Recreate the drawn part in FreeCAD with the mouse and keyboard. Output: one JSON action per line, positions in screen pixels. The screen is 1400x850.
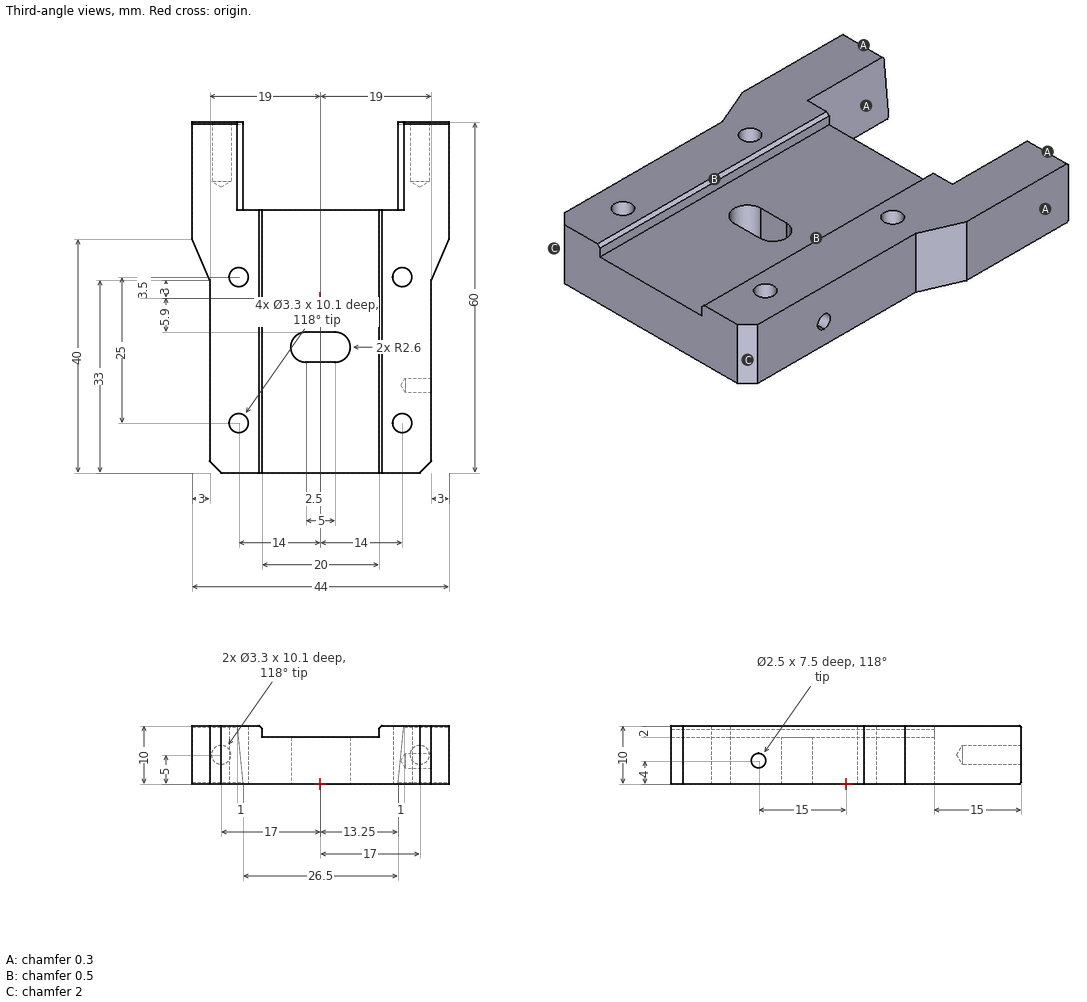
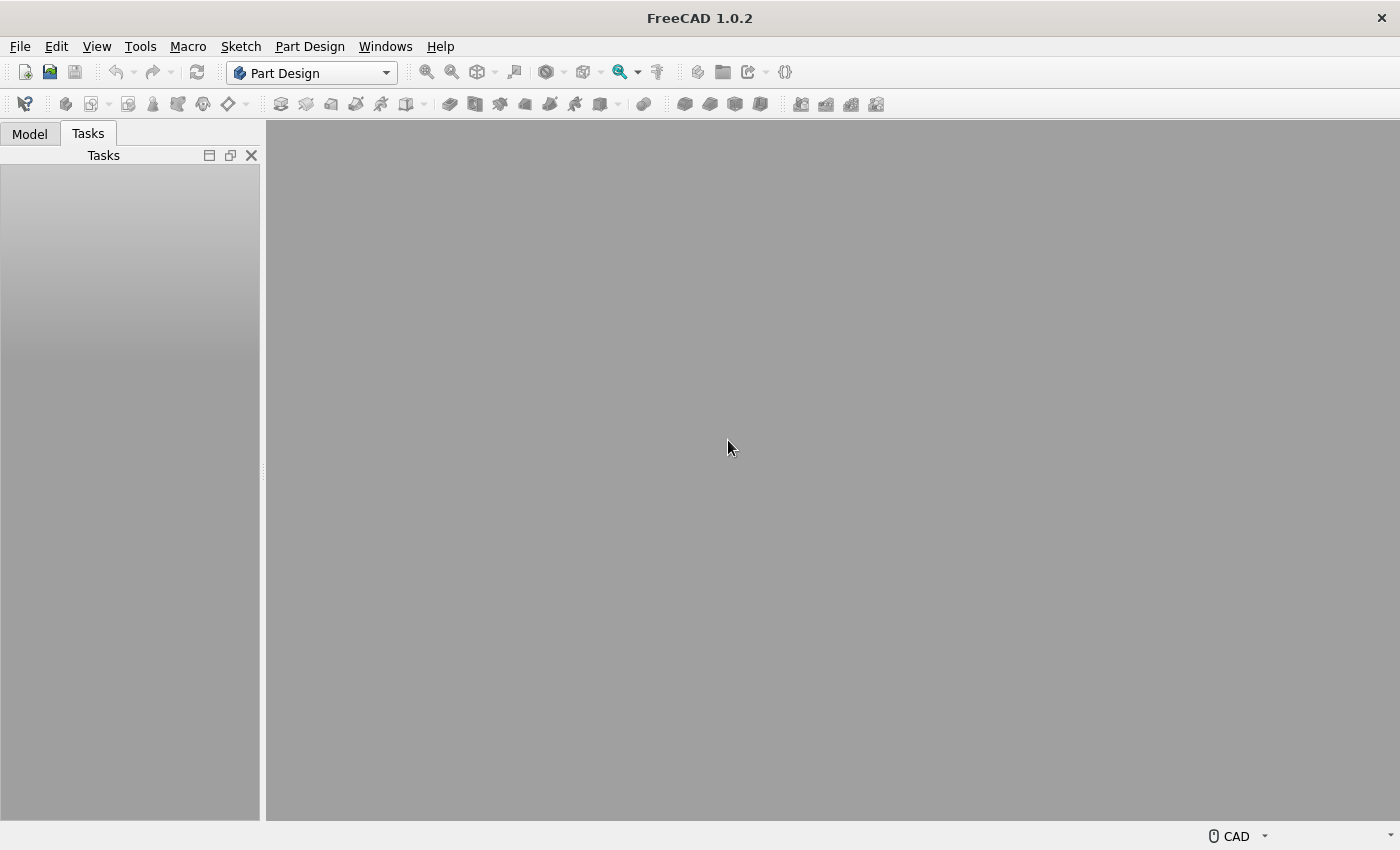
{"action": "key", "text": "ctrl+n"}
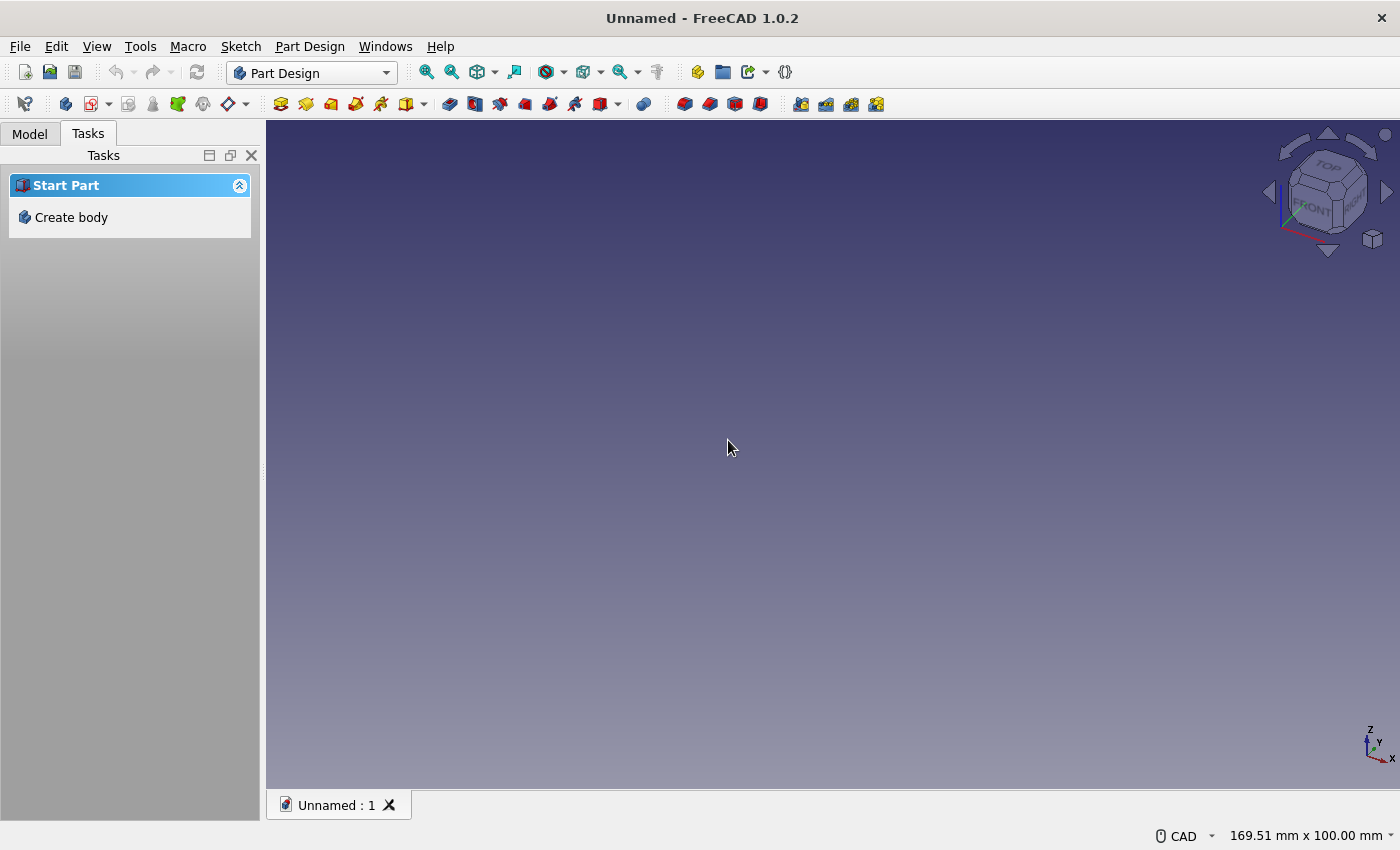
{"action": "left_click", "coordinate": [90, 104]}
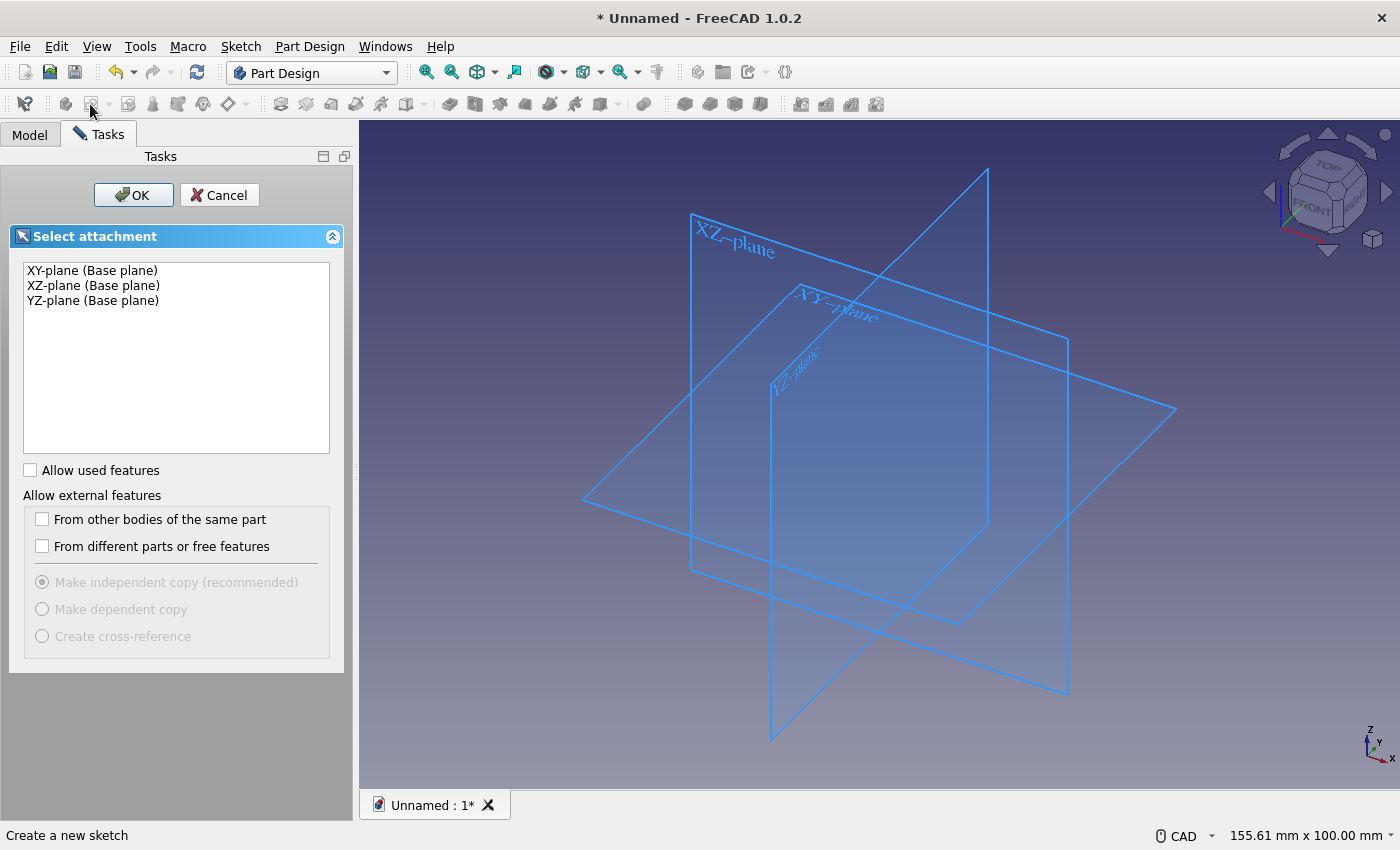
{"action": "left_click", "coordinate": [84, 270]}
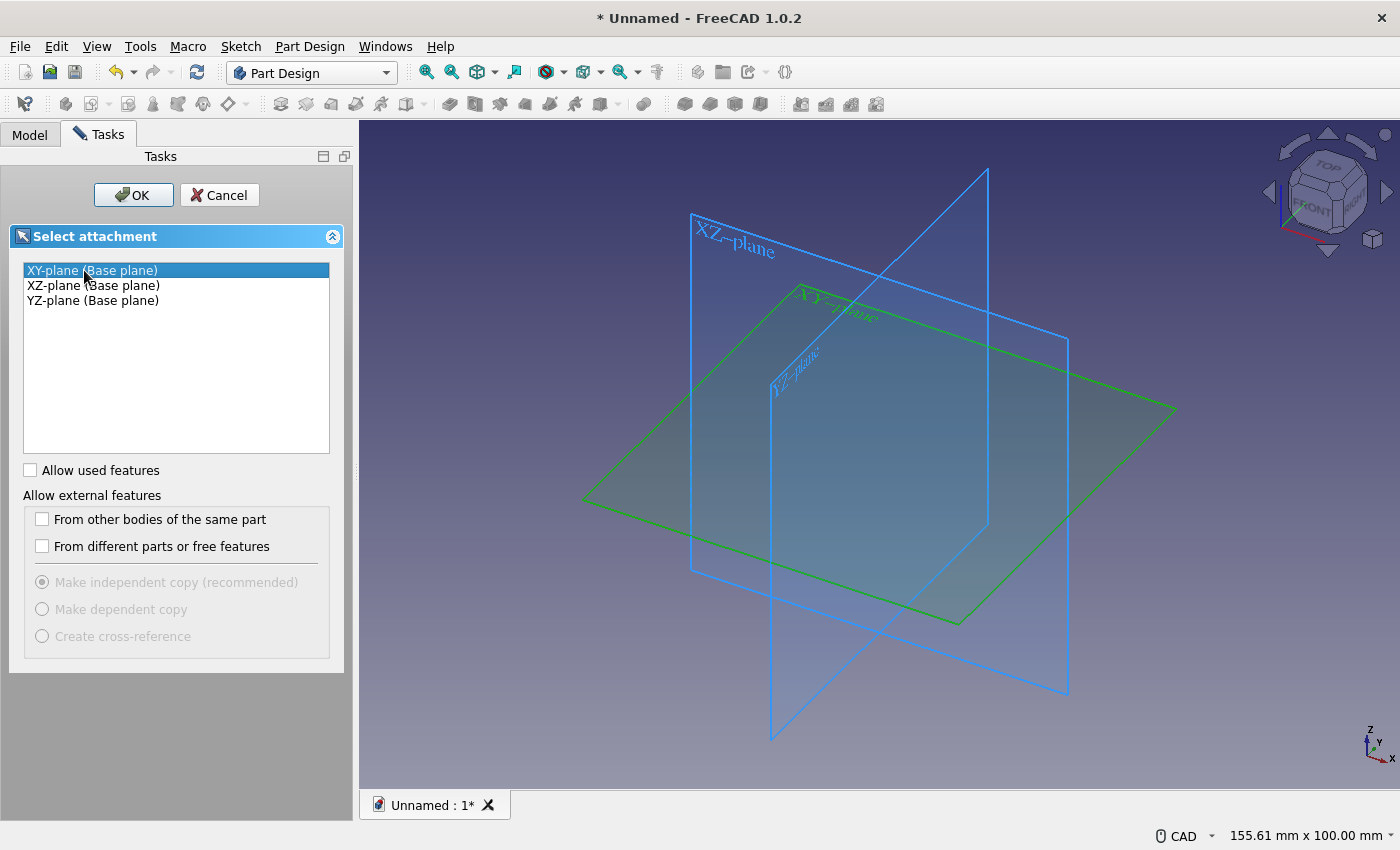
{"action": "left_click", "coordinate": [134, 195]}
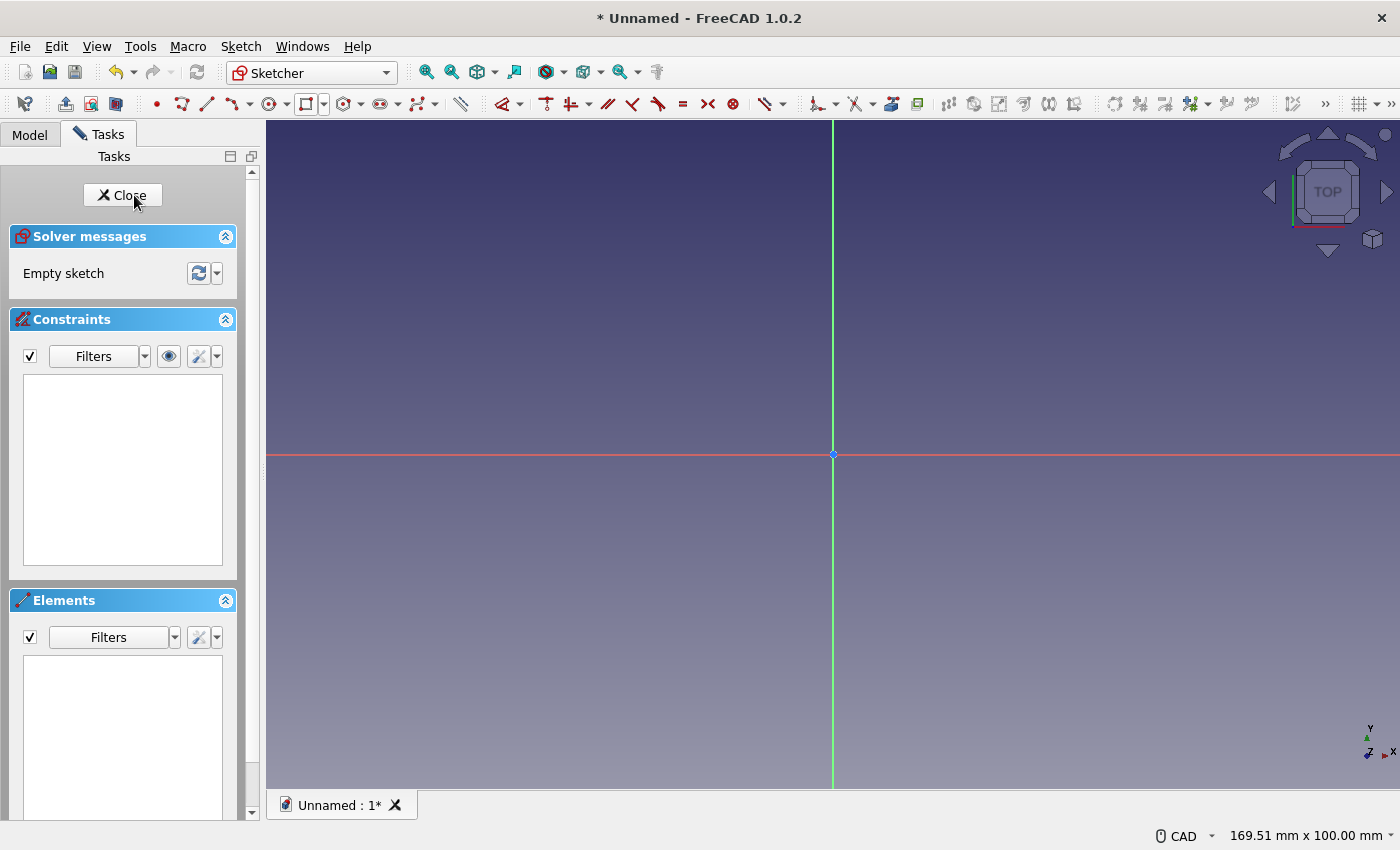
{"action": "left_click", "coordinate": [324, 104]}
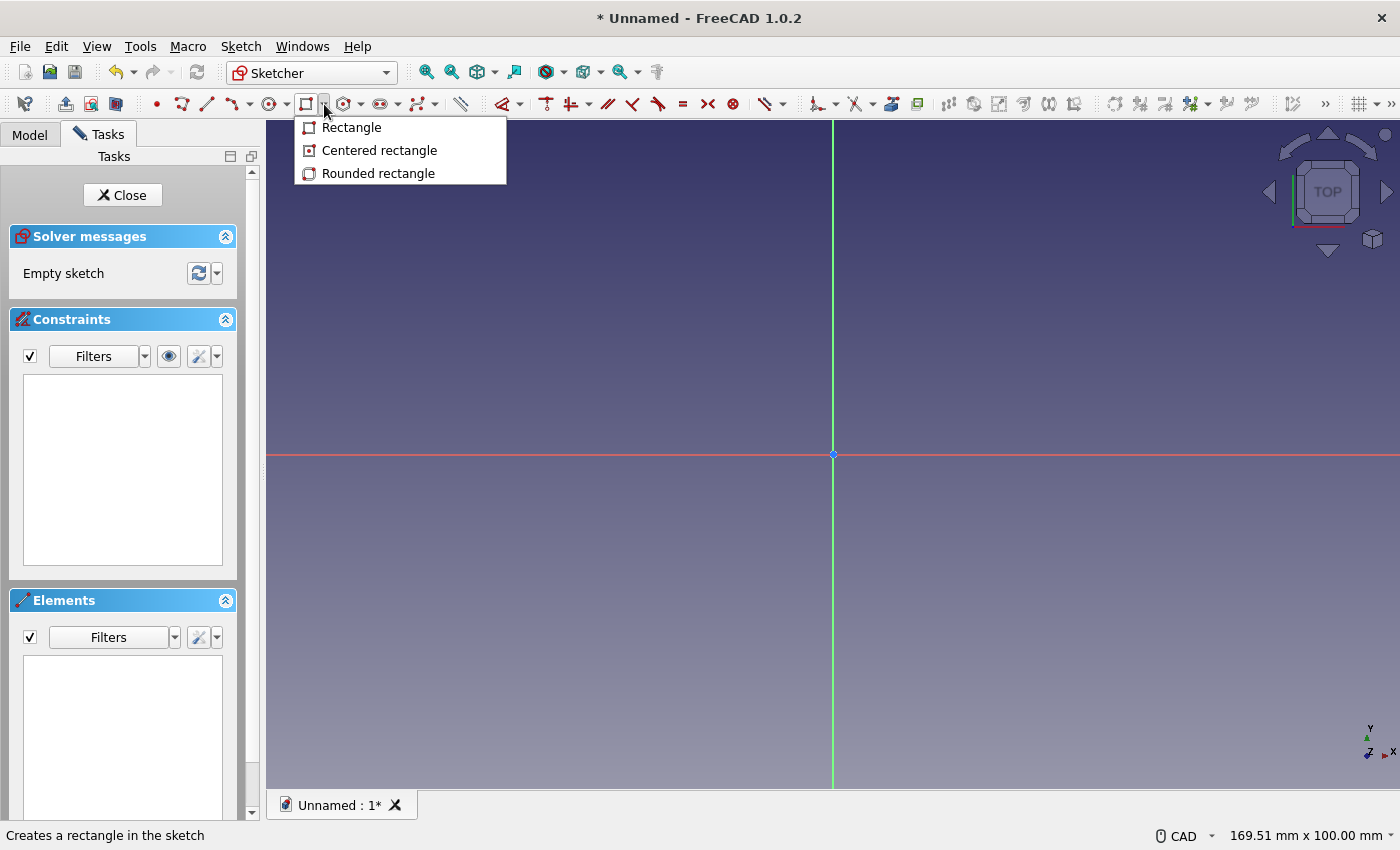
{"action": "left_click", "coordinate": [400, 150]}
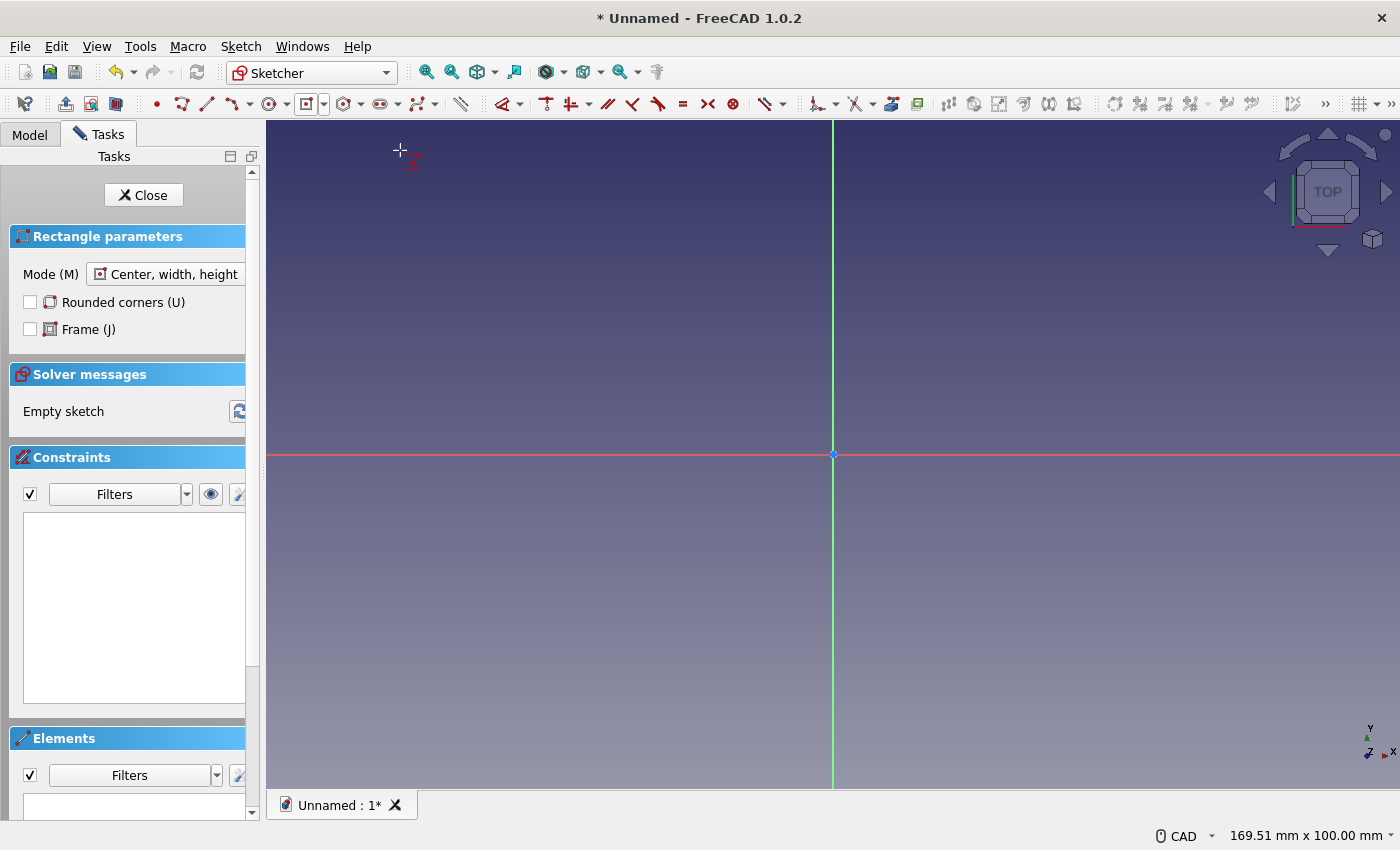
{"action": "left_click", "coordinate": [833, 454]}
{"action": "left_click", "coordinate": [980, 254]}
{"action": "key", "text": "Escape"}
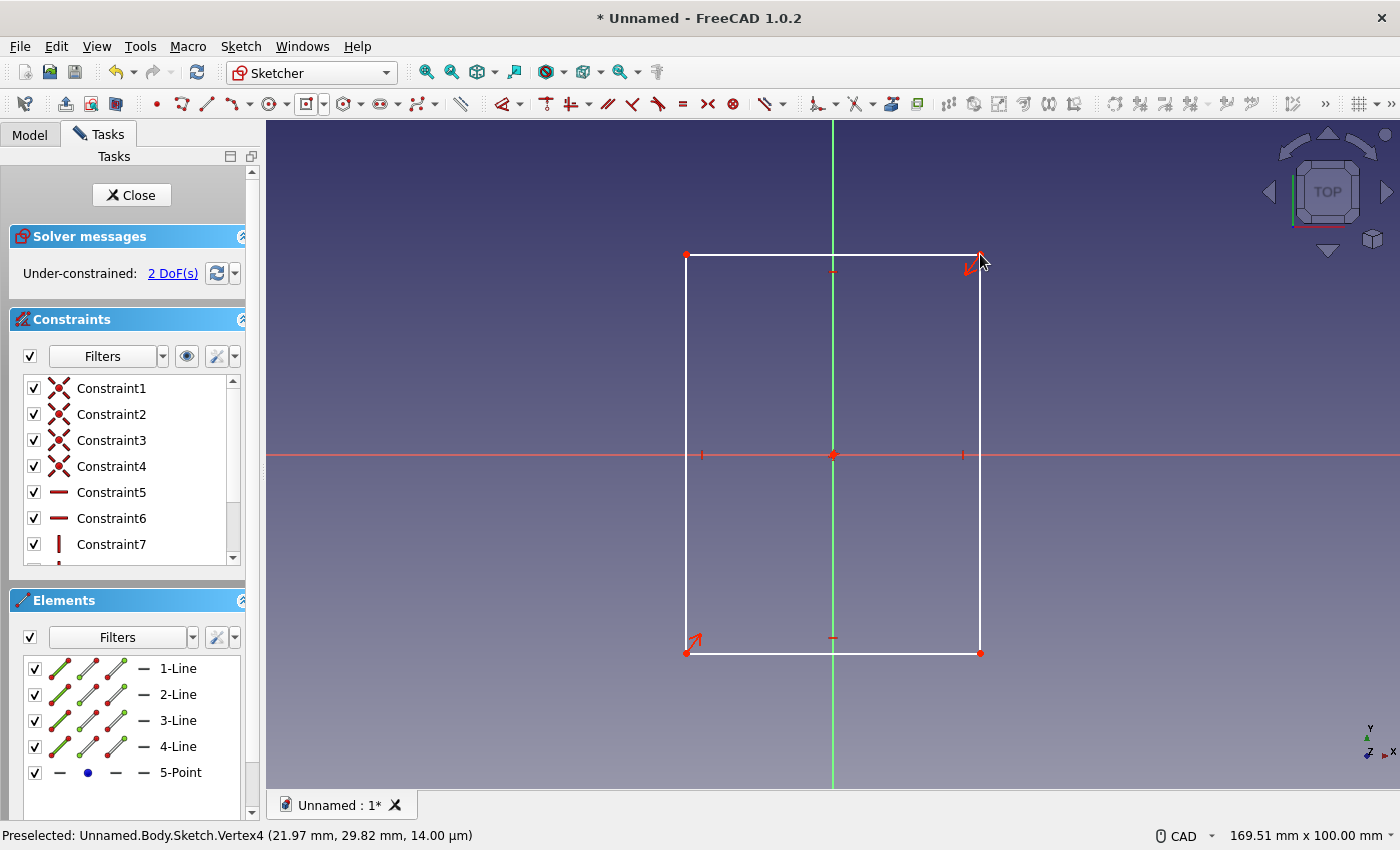
{"action": "left_click", "coordinate": [774, 654]}